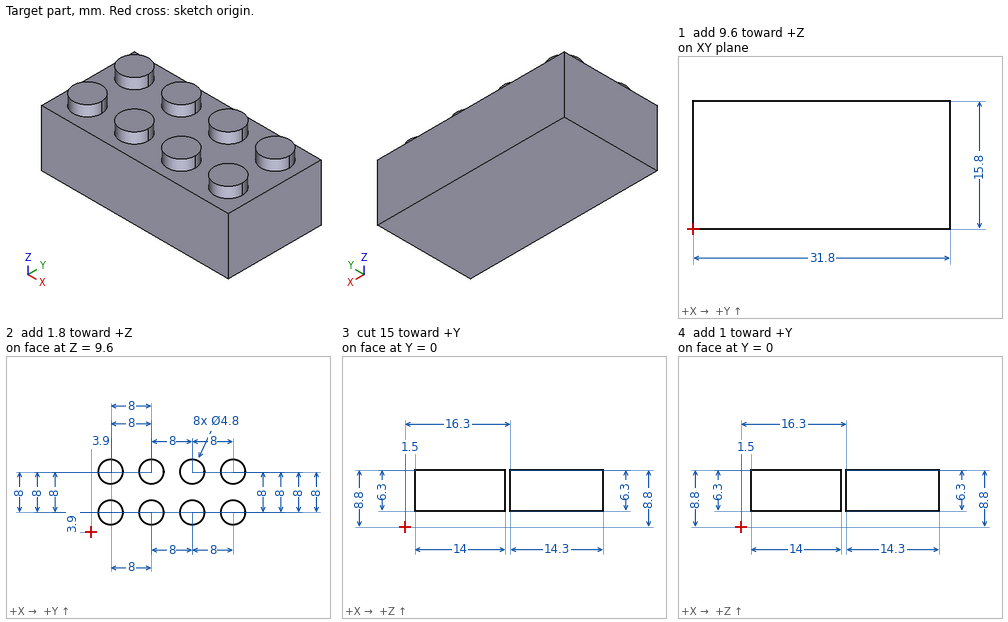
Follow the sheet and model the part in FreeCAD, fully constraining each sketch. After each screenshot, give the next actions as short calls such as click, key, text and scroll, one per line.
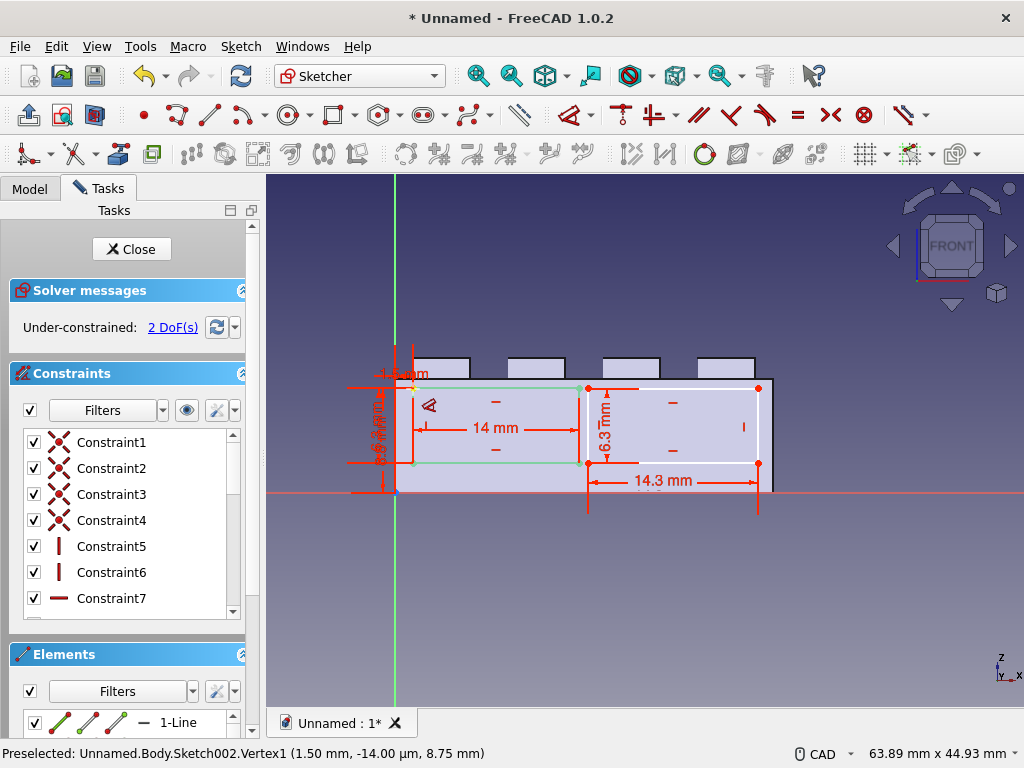
scroll(588, 389, up, 2)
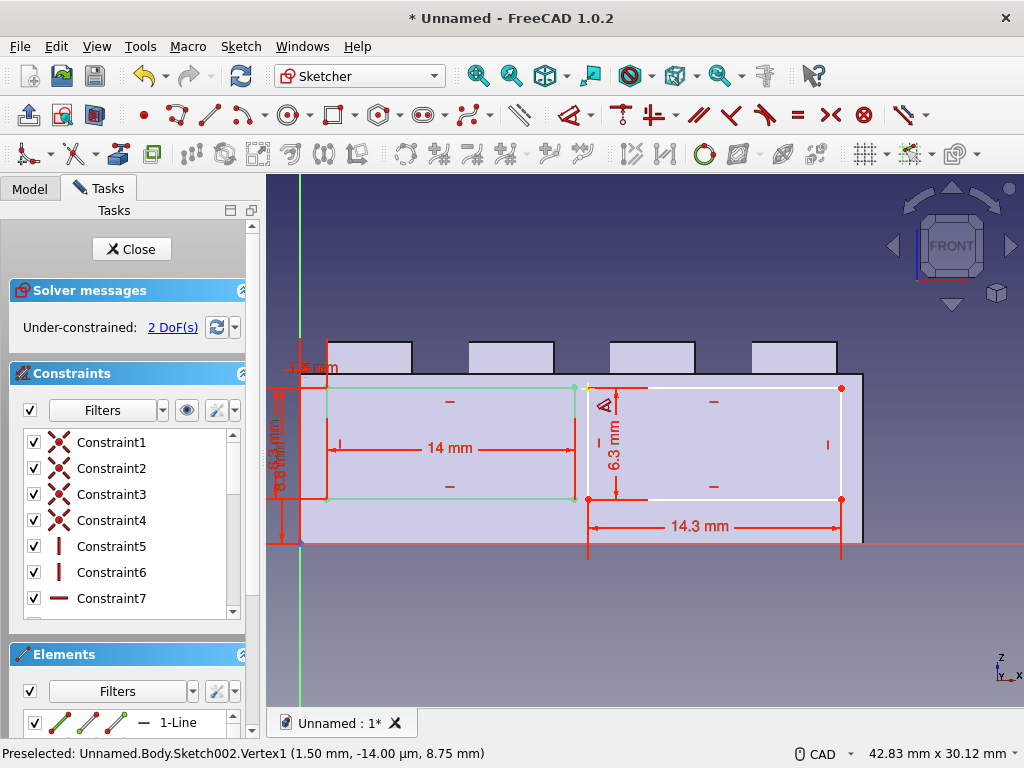
click(588, 388)
click(622, 466)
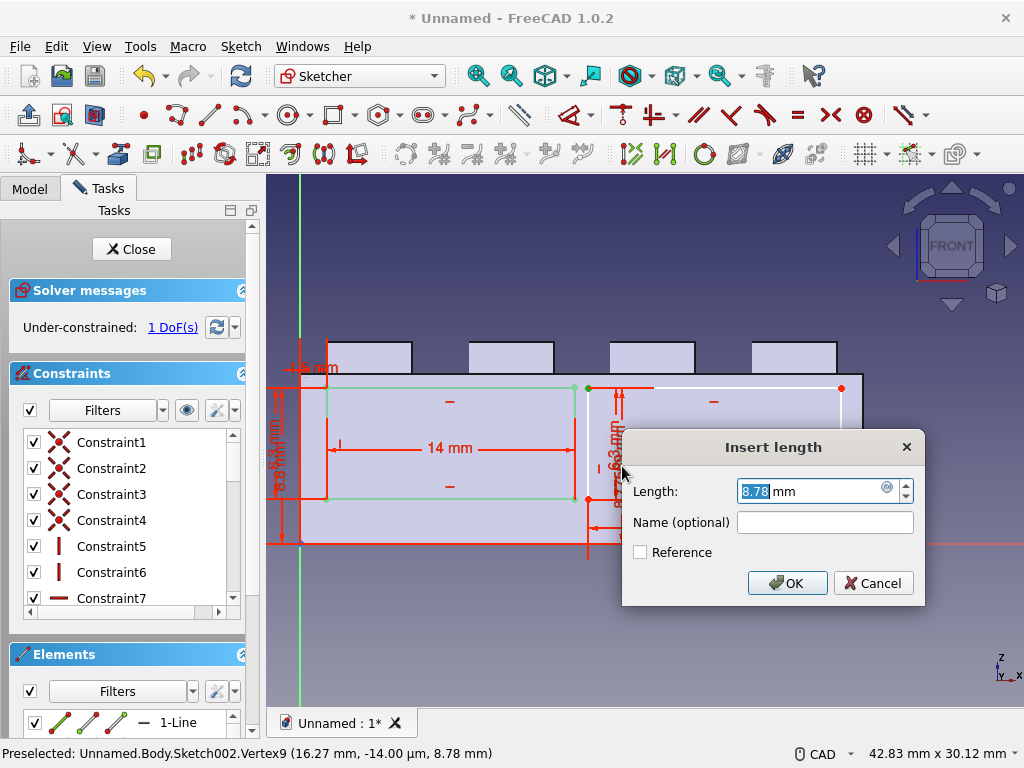
text(8.8)
key(Return)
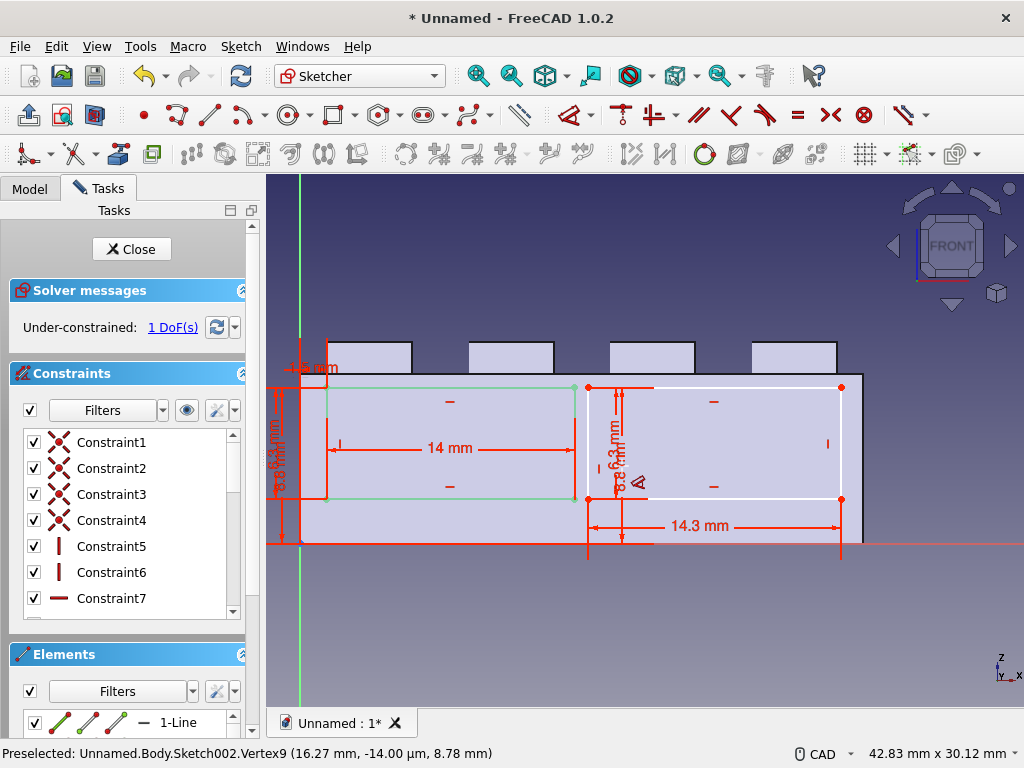
click(588, 388)
click(444, 578)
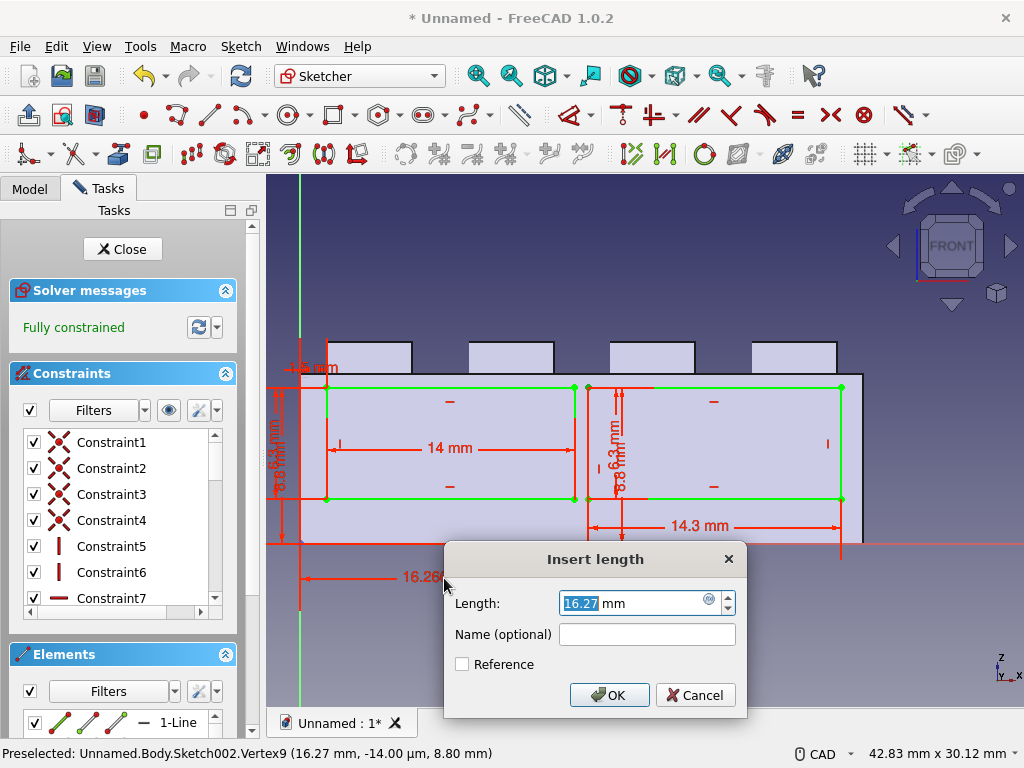
text(16.3)
key(Return)
key(Escape)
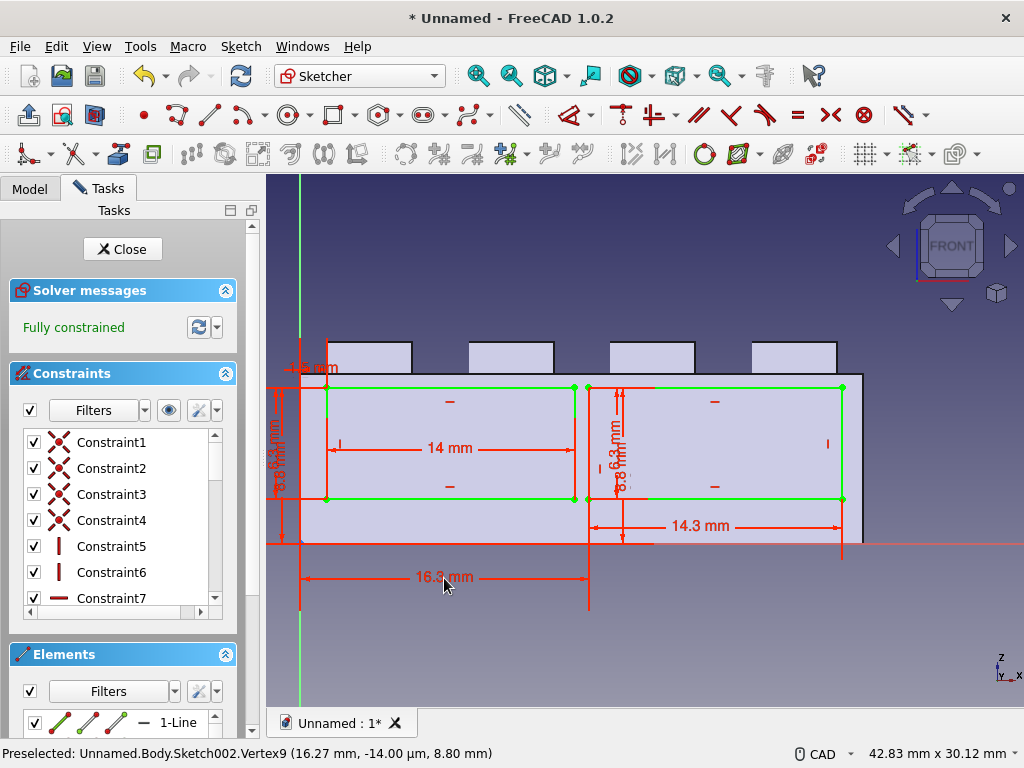
click(123, 249)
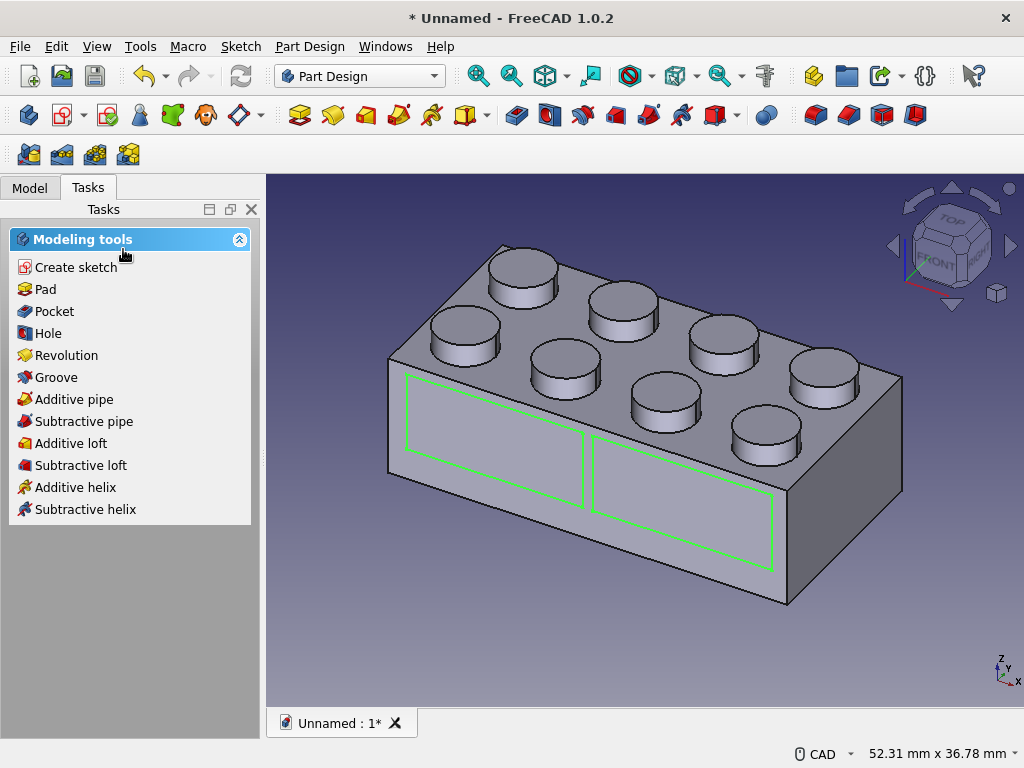
click(517, 116)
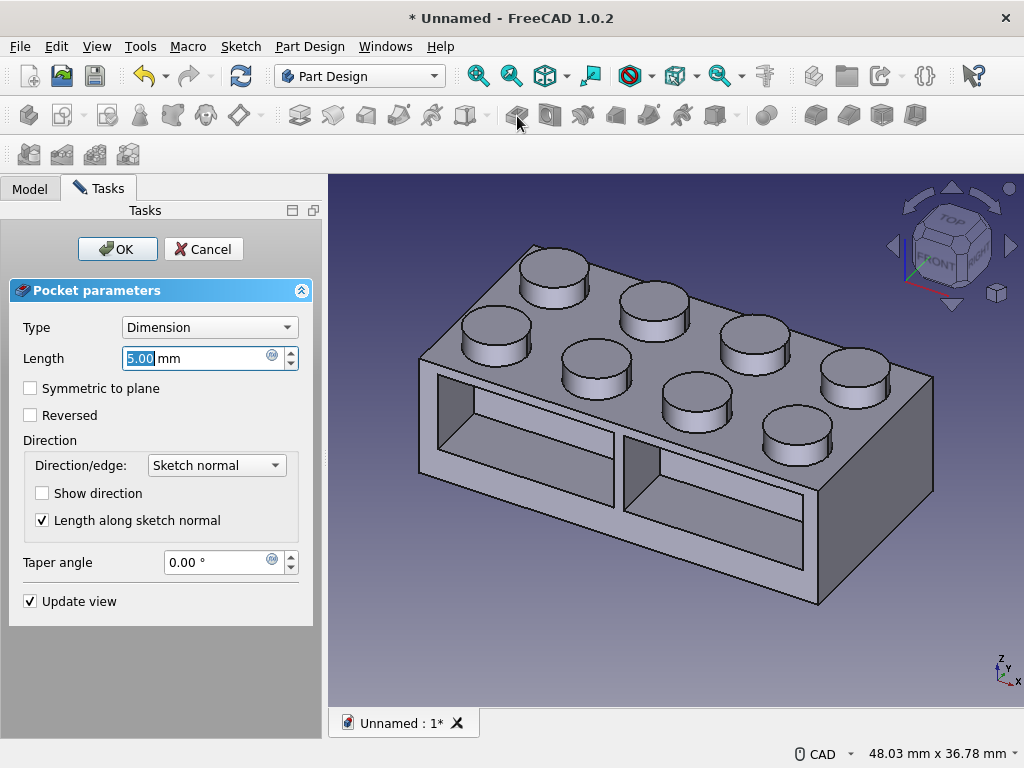
text(15)
key(Tab)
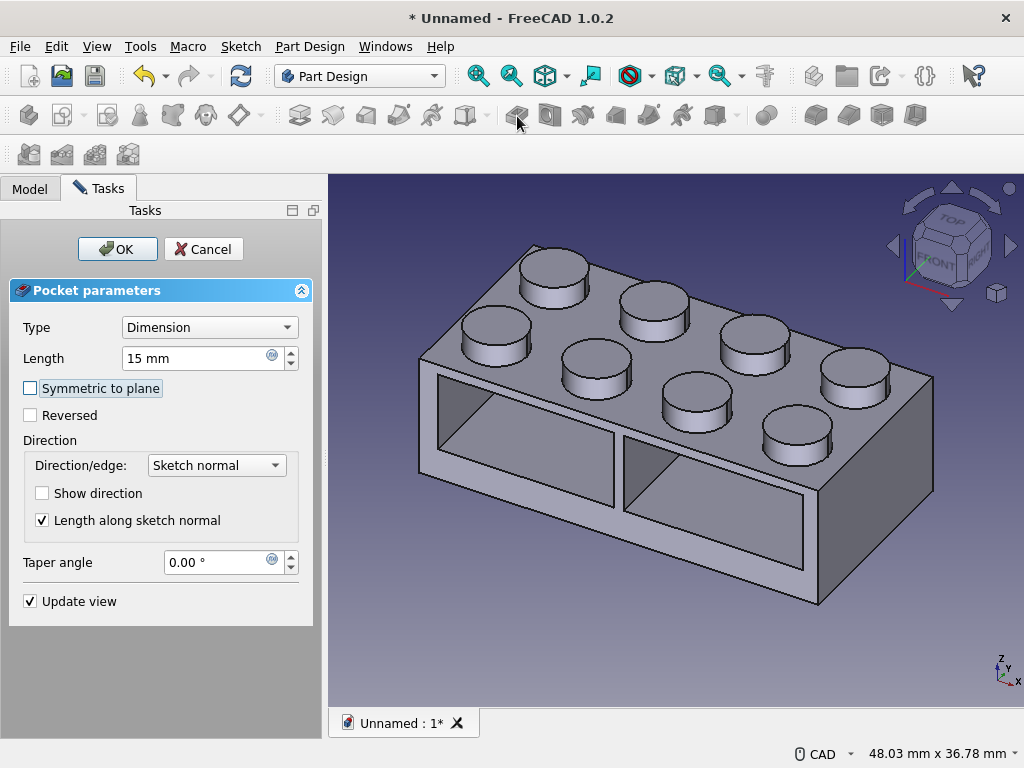
click(118, 249)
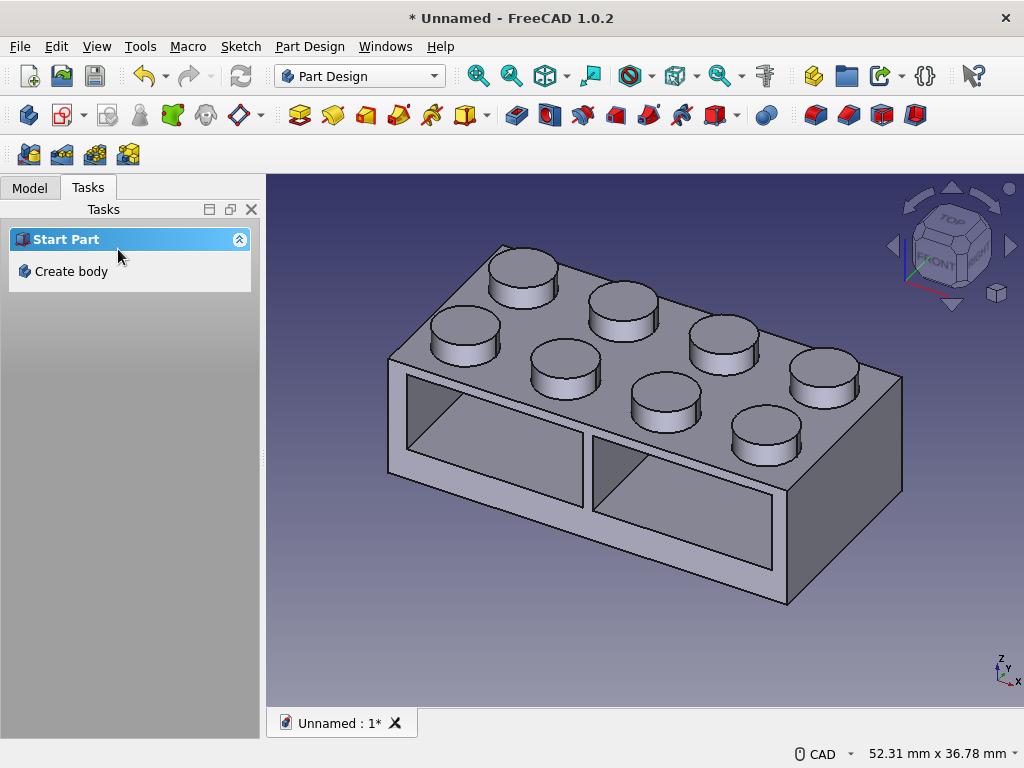
click(759, 586)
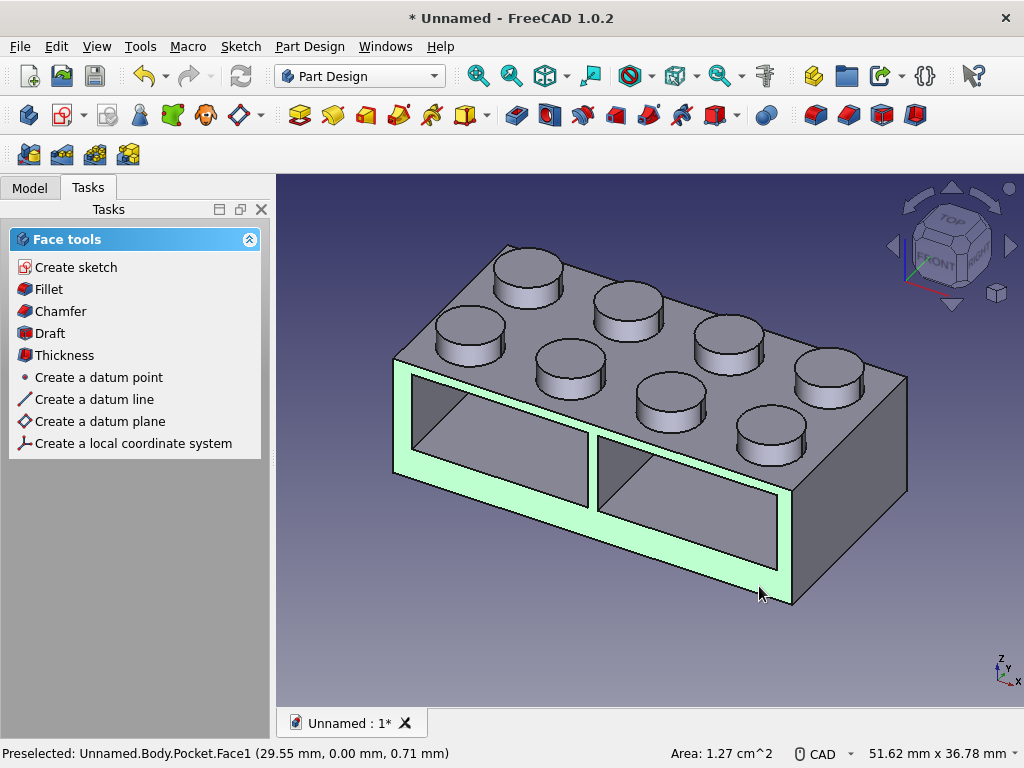
click(62, 116)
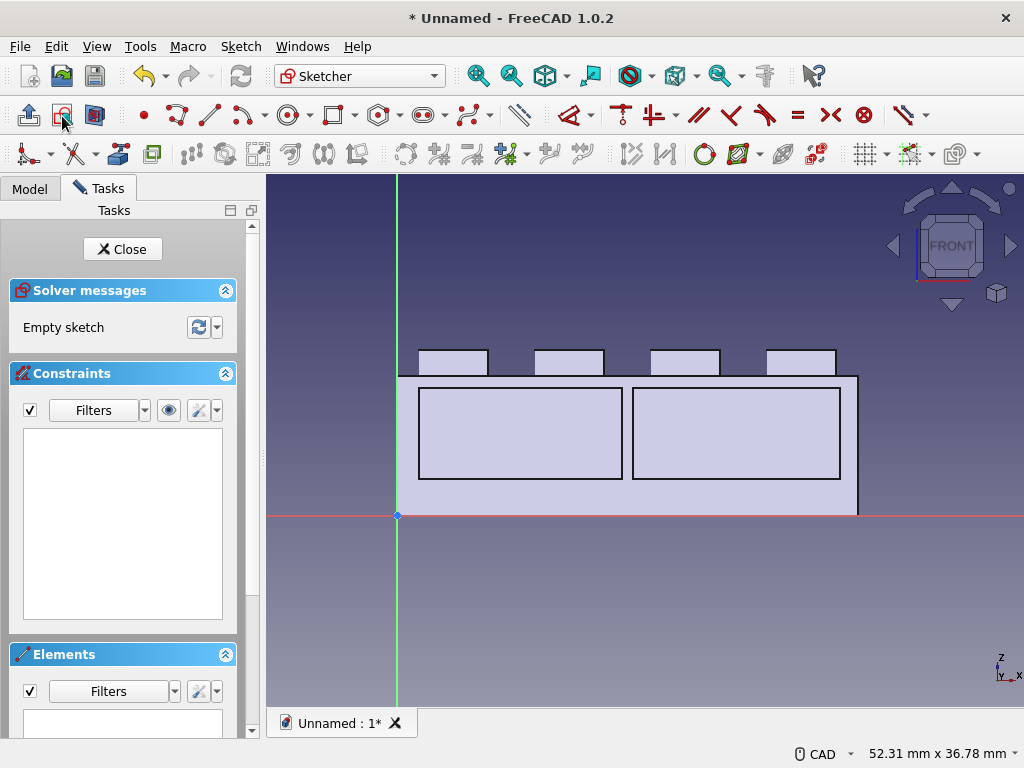
scroll(385, 390, down, 1)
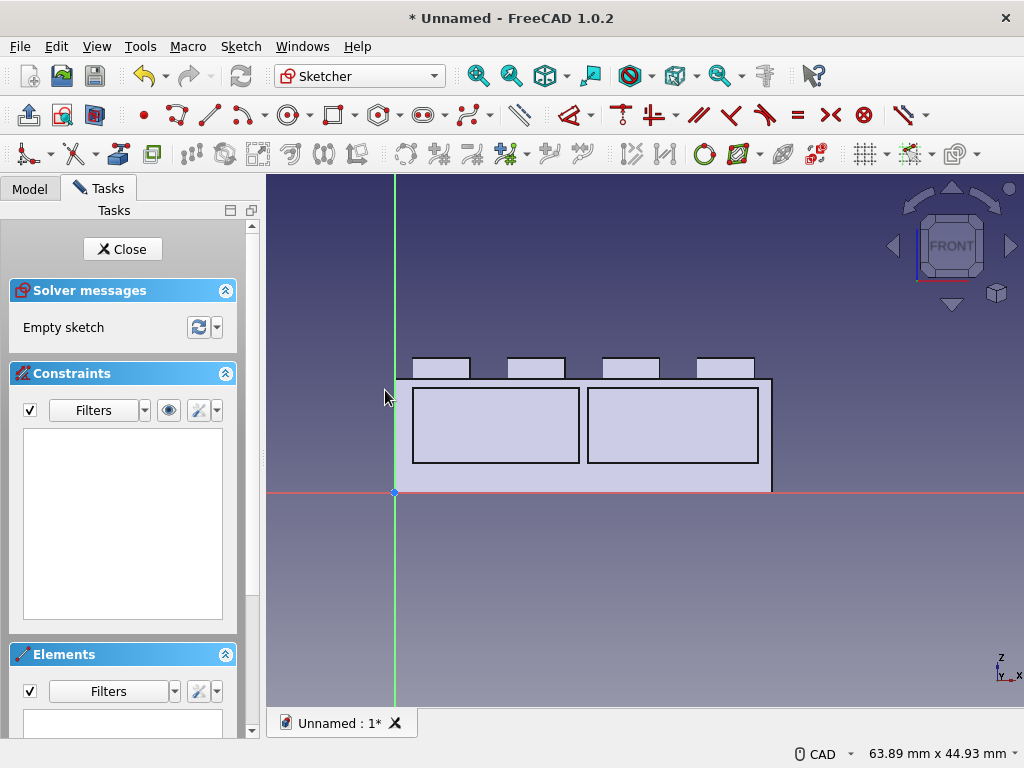
key(g)
key(r)